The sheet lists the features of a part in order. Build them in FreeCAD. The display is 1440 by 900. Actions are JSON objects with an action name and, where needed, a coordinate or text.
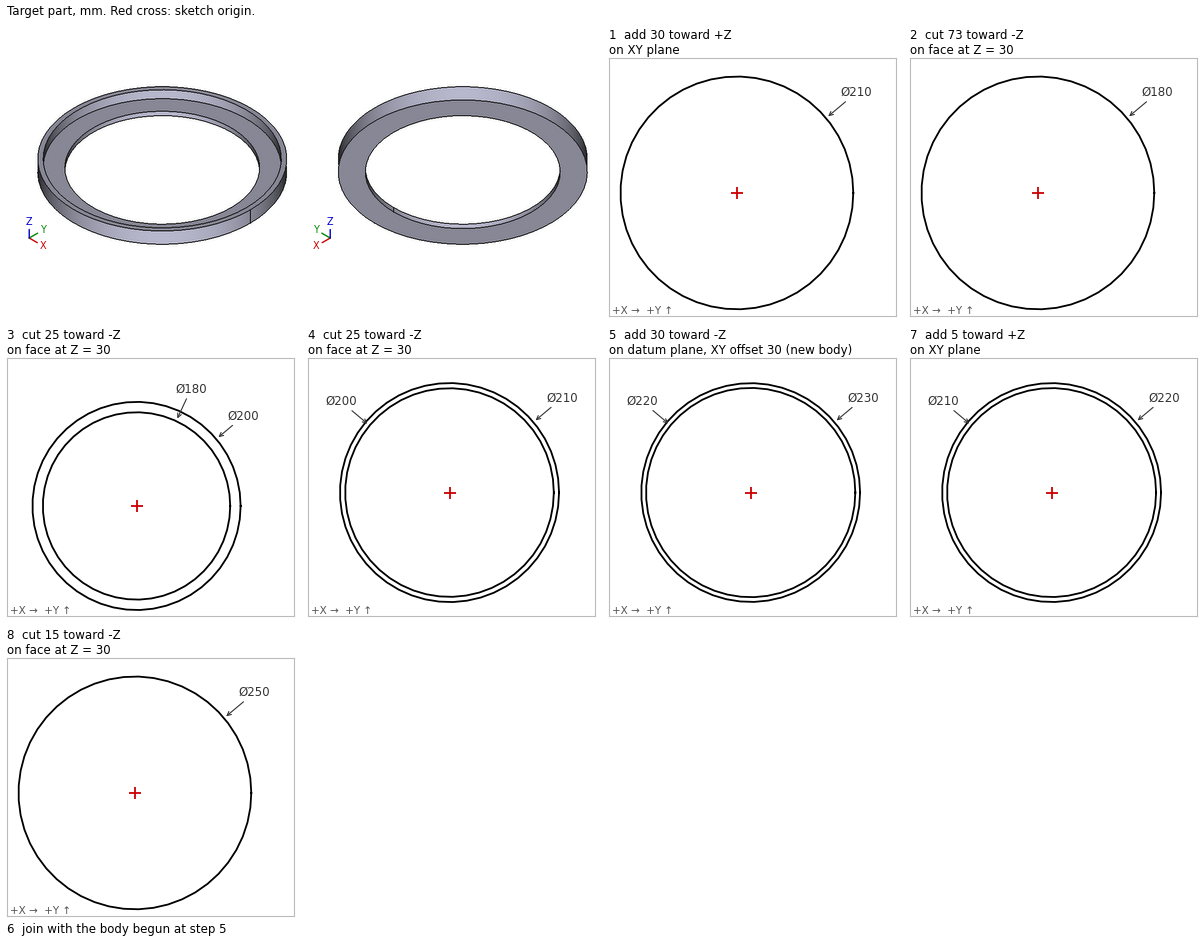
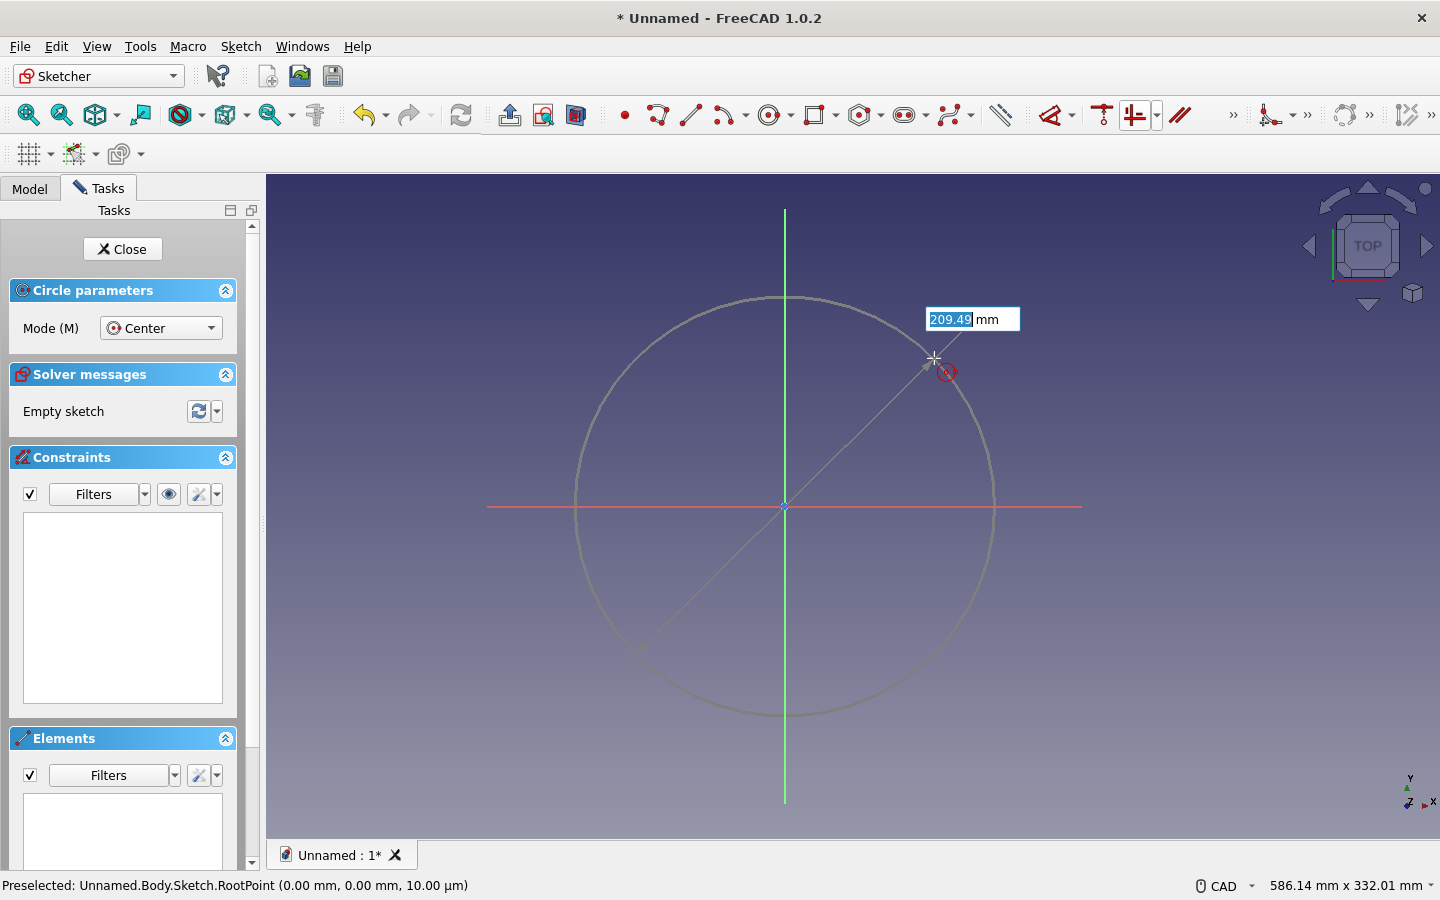
{"action": "type", "text": "210"}
{"action": "key", "text": "Return"}
{"action": "key", "text": "Escape"}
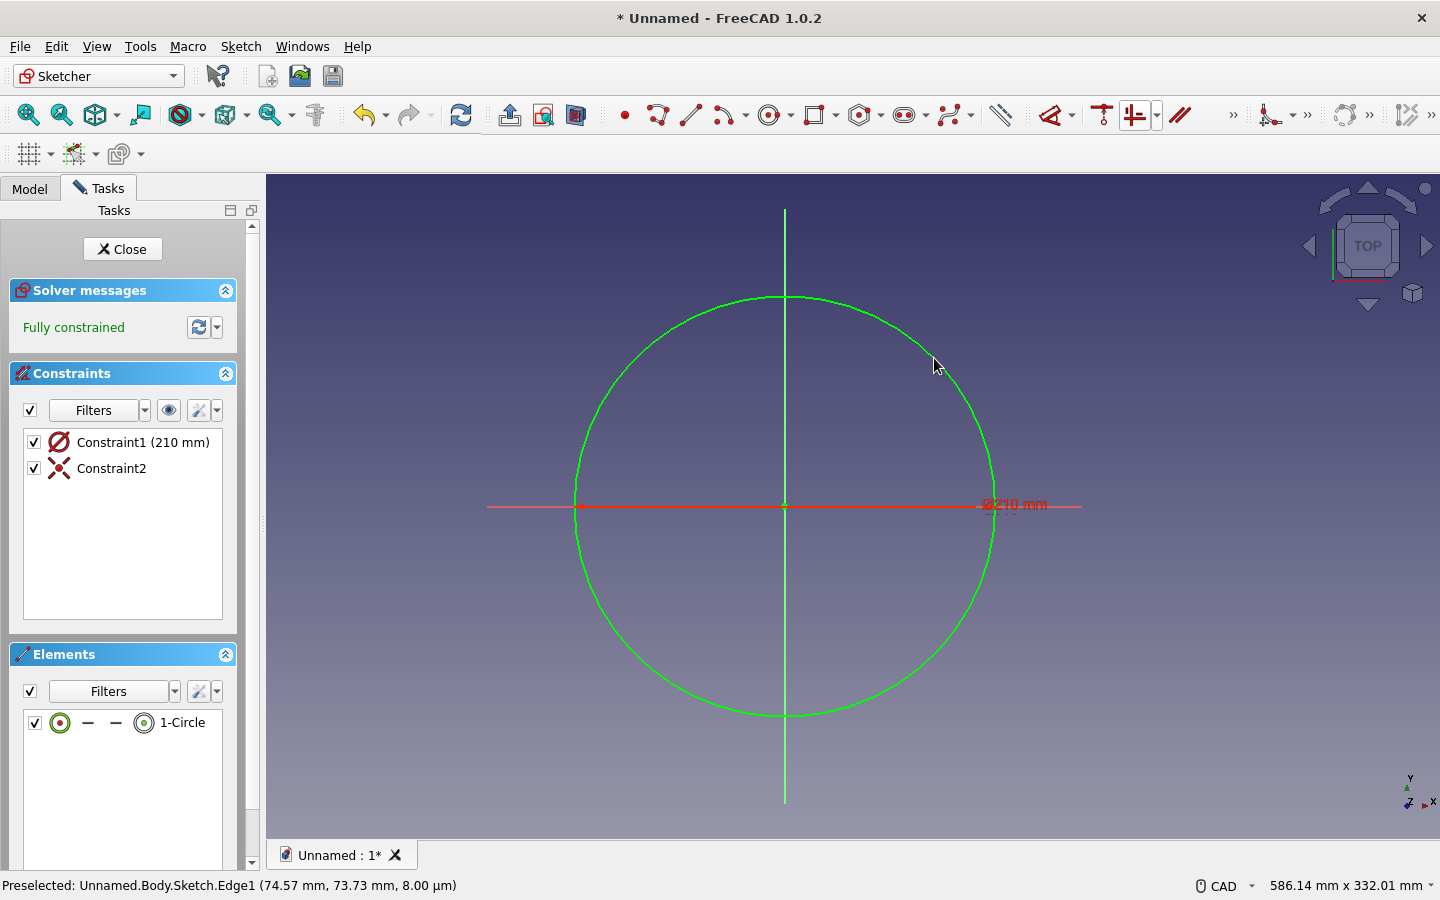
{"action": "left_click", "coordinate": [123, 249]}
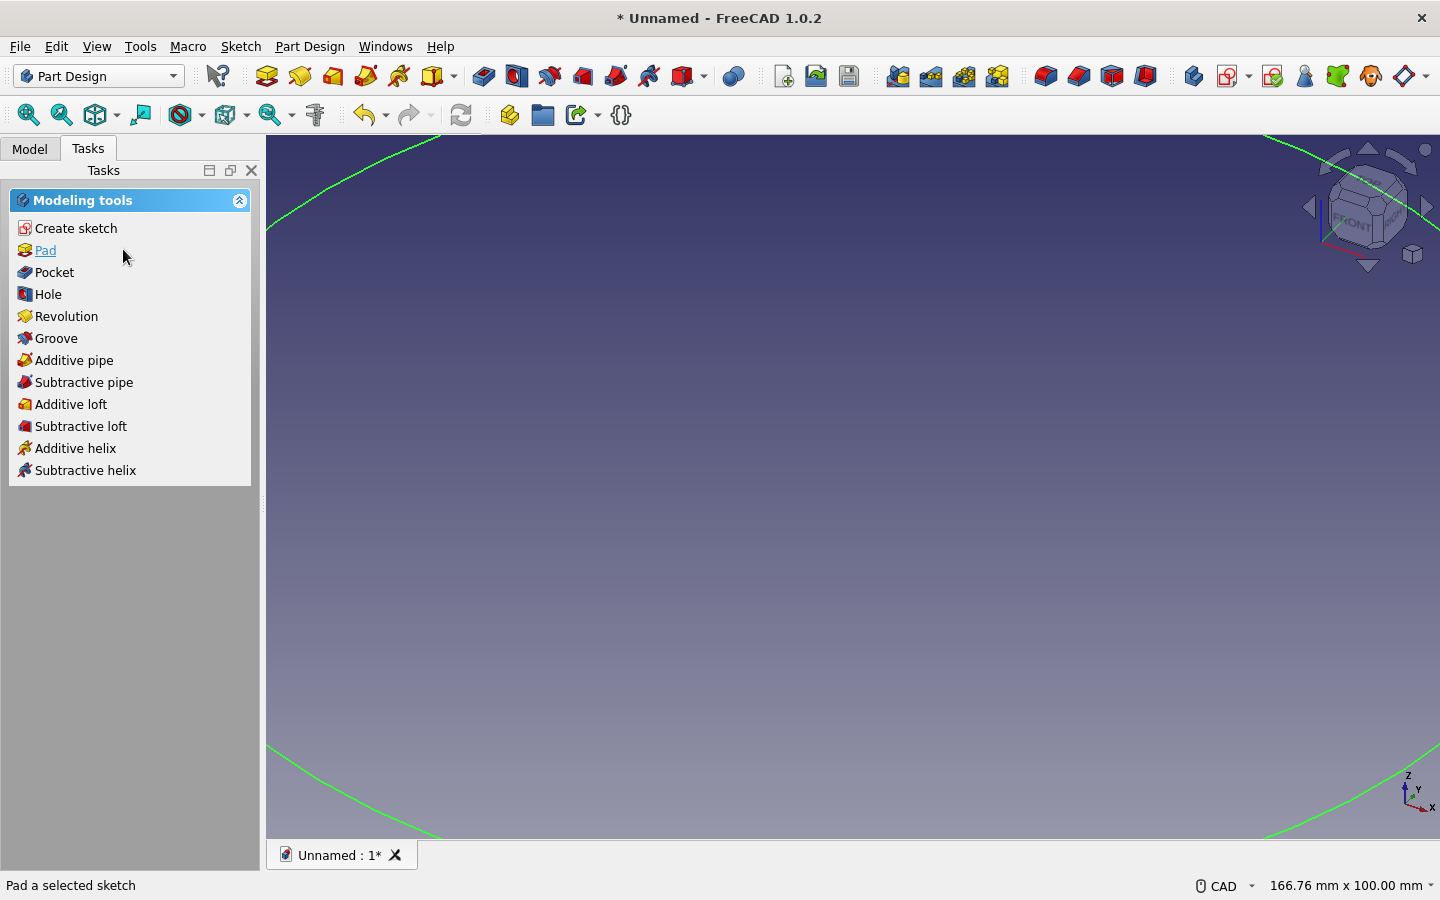
{"action": "left_click", "coordinate": [267, 76]}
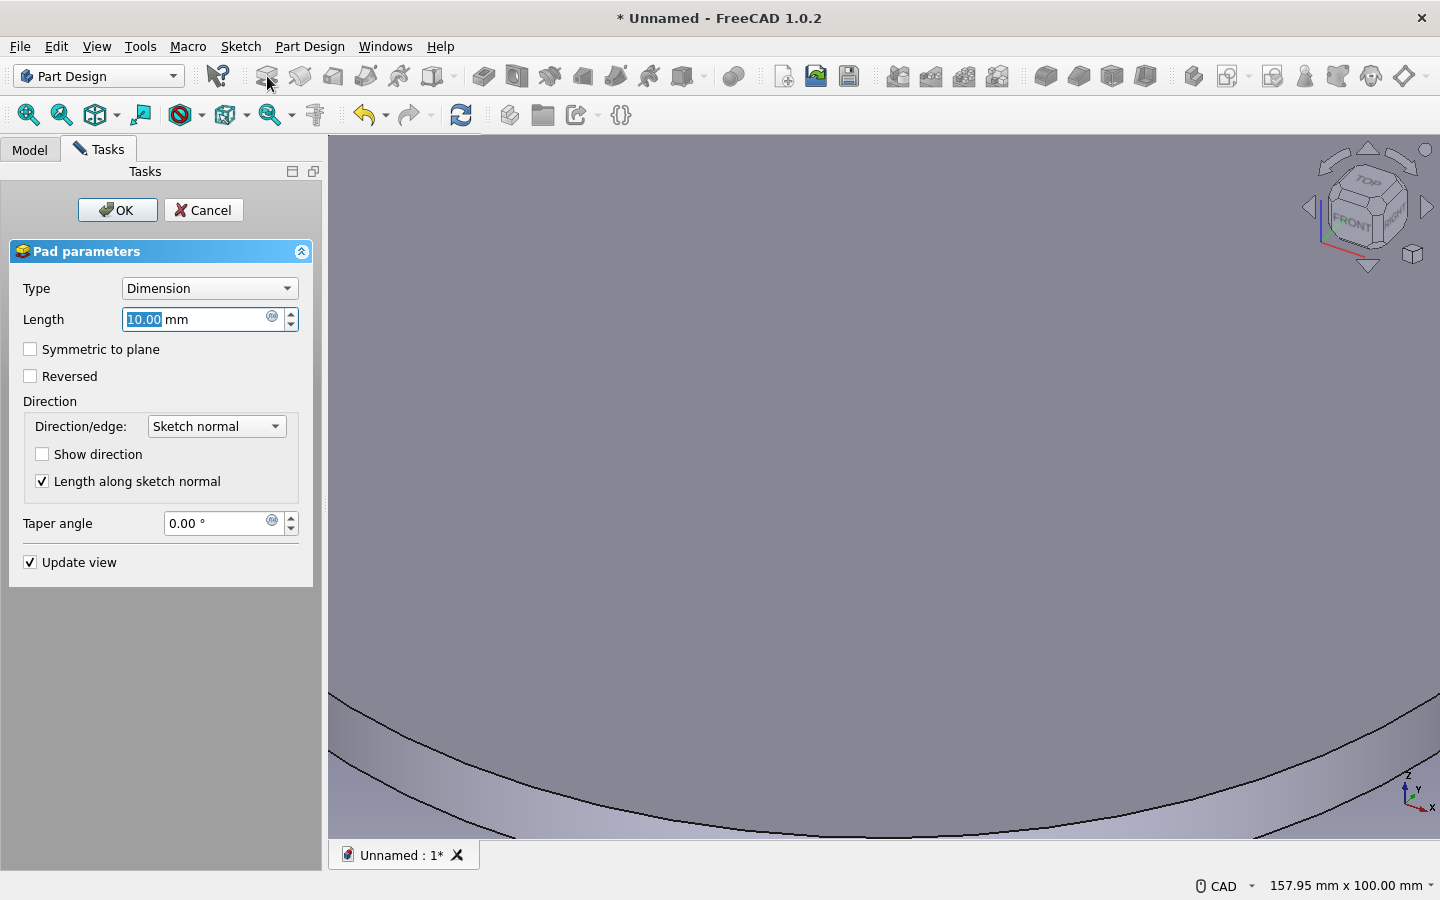
{"action": "type", "text": "30"}
{"action": "key", "text": "Tab"}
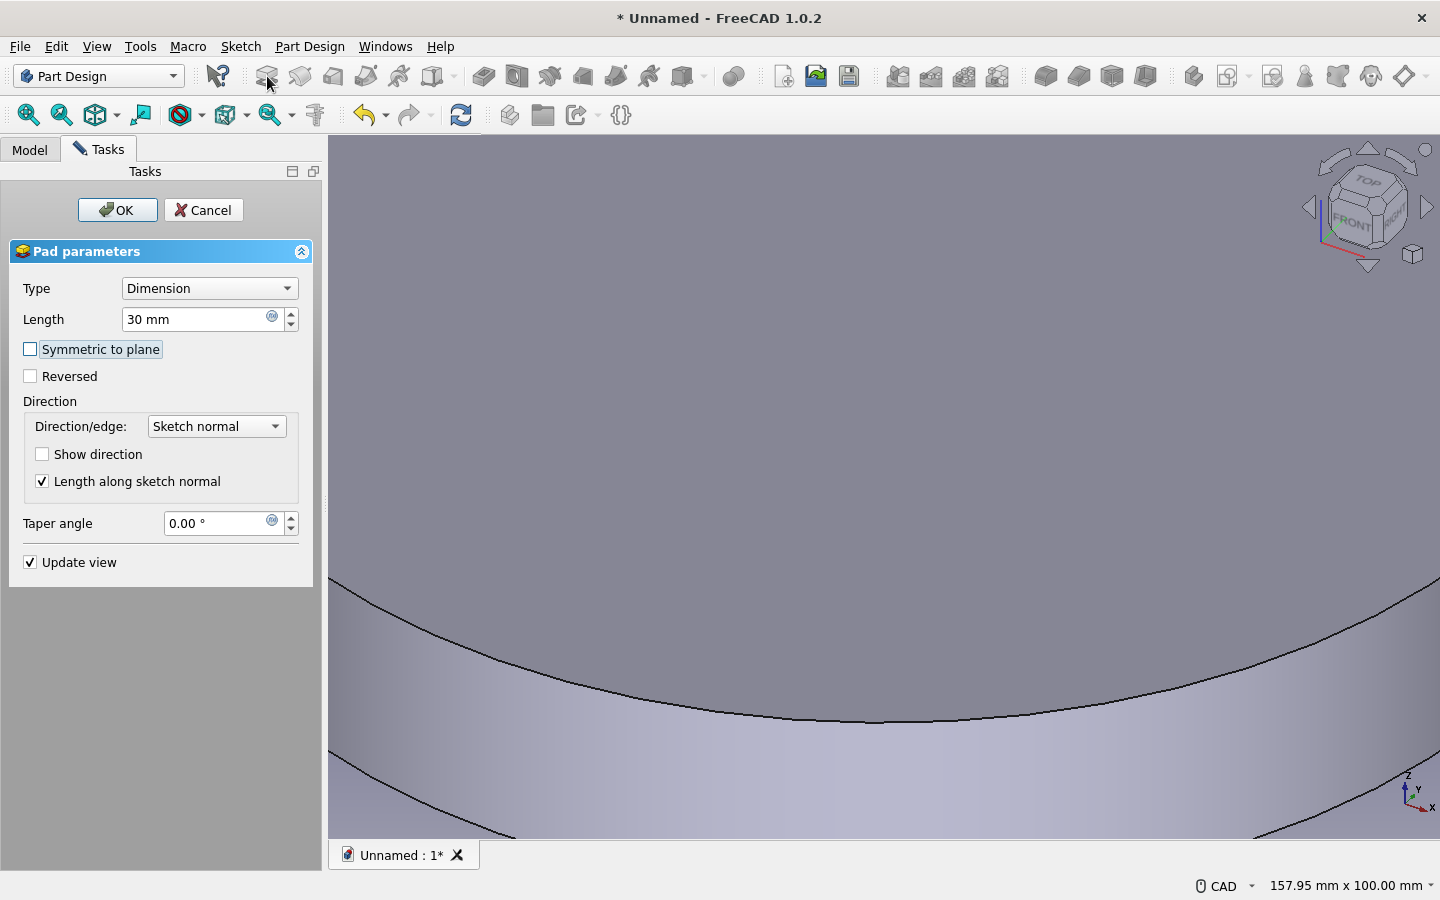
{"action": "left_click", "coordinate": [118, 210]}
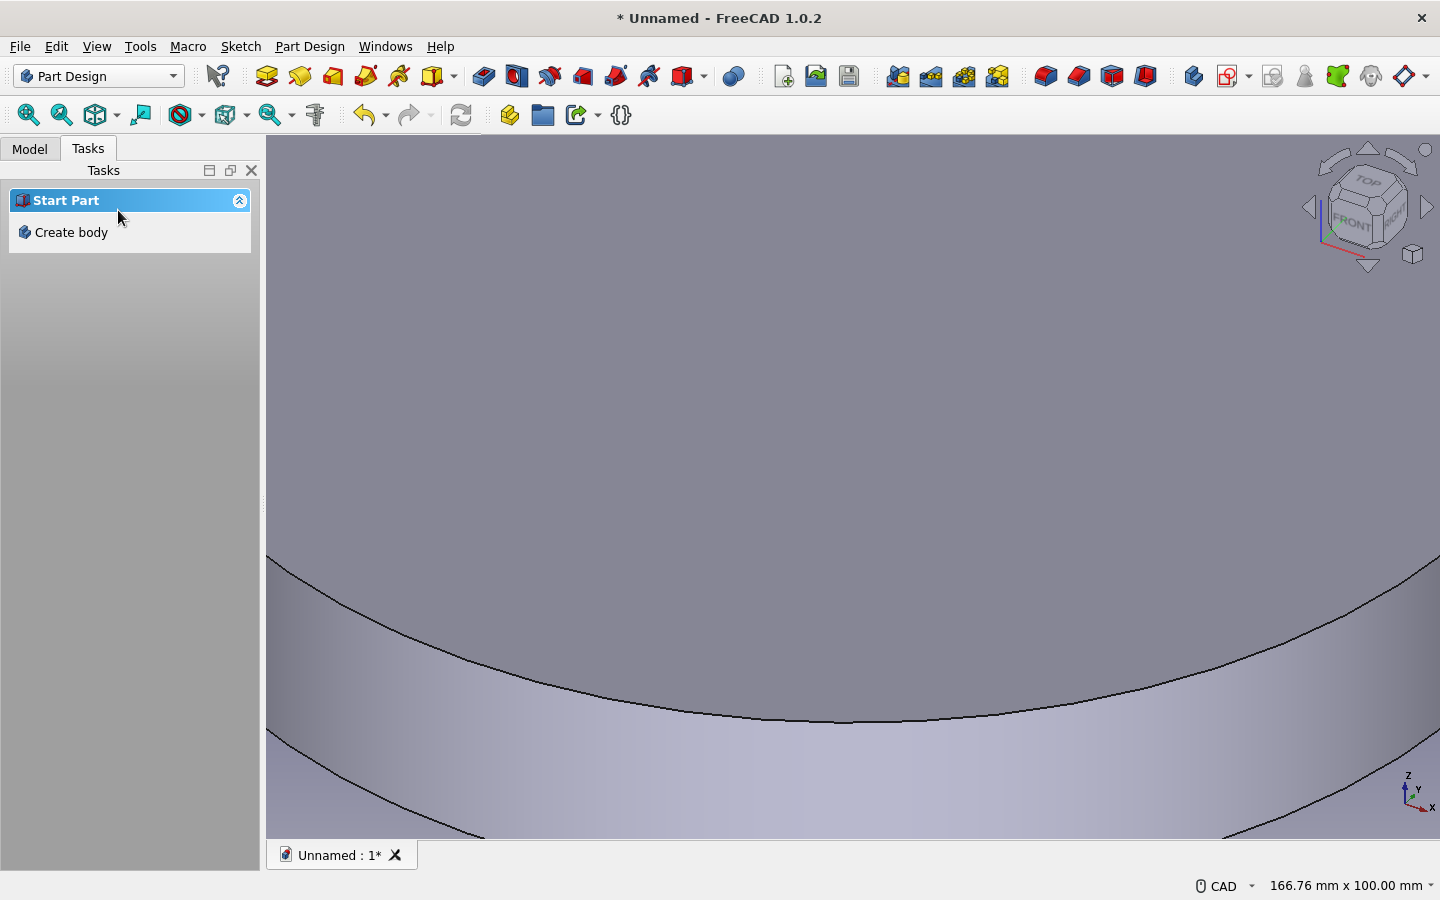
{"action": "left_click", "coordinate": [29, 116]}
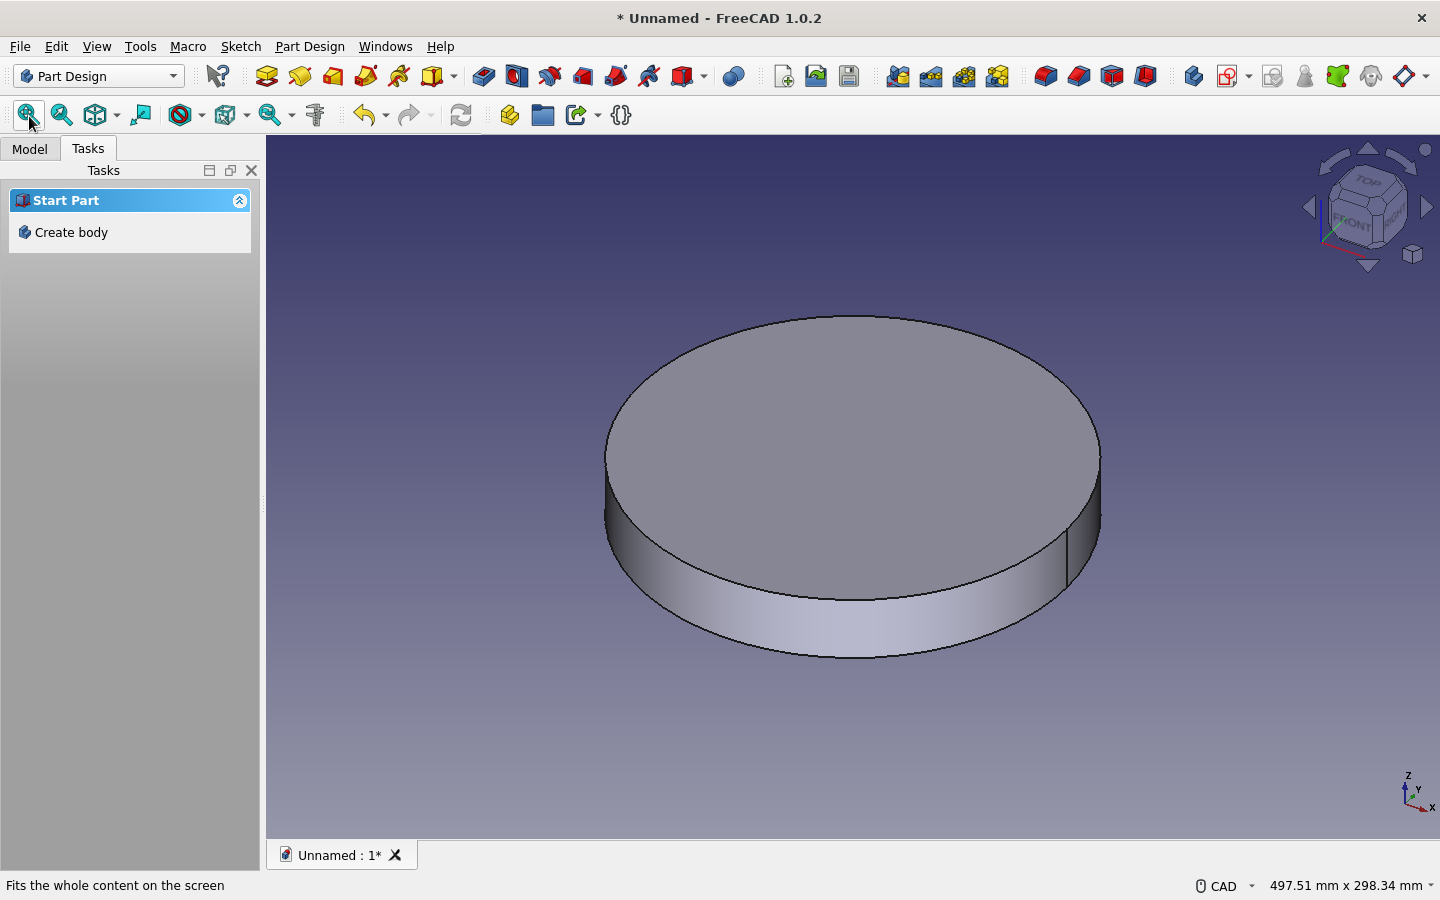
{"action": "left_click", "coordinate": [853, 457]}